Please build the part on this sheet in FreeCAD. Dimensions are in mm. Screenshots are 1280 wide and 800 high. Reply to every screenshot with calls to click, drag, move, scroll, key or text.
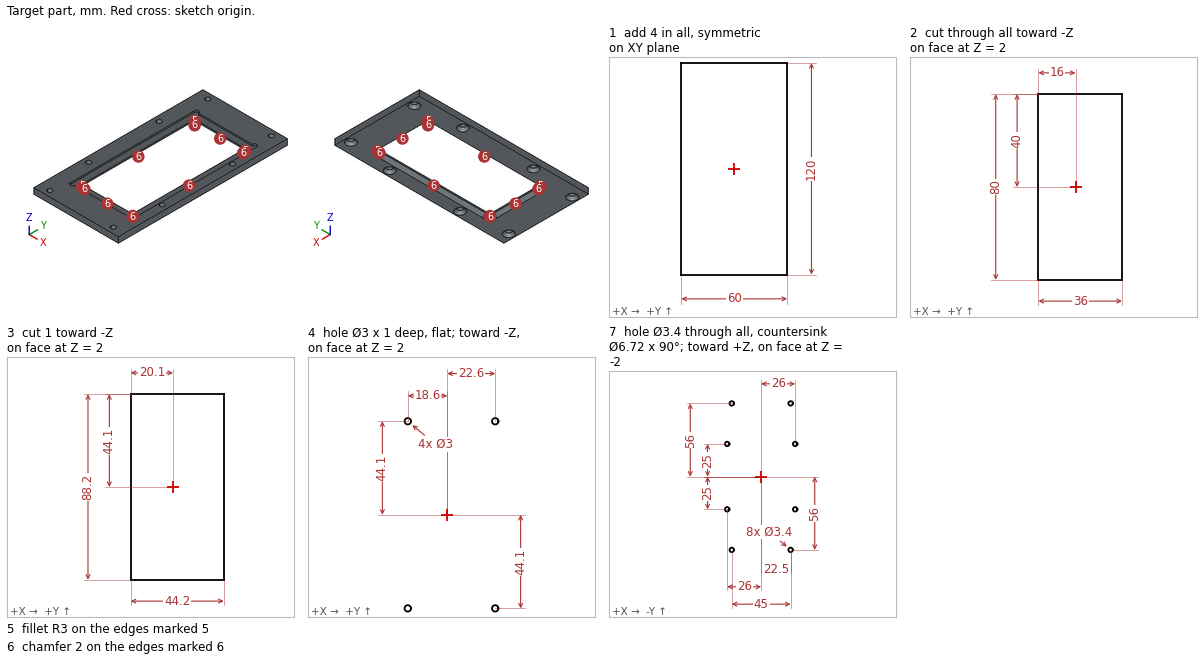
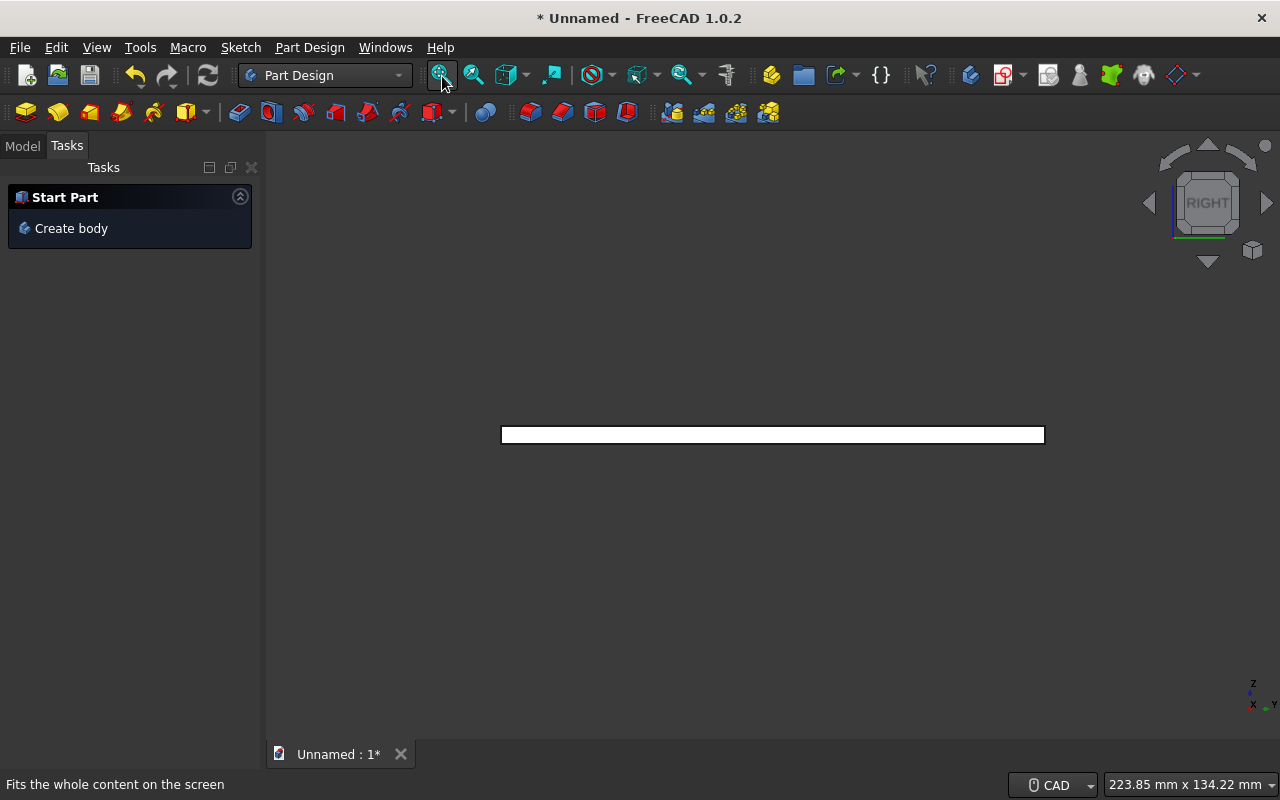
scroll(592, 436, up, 6)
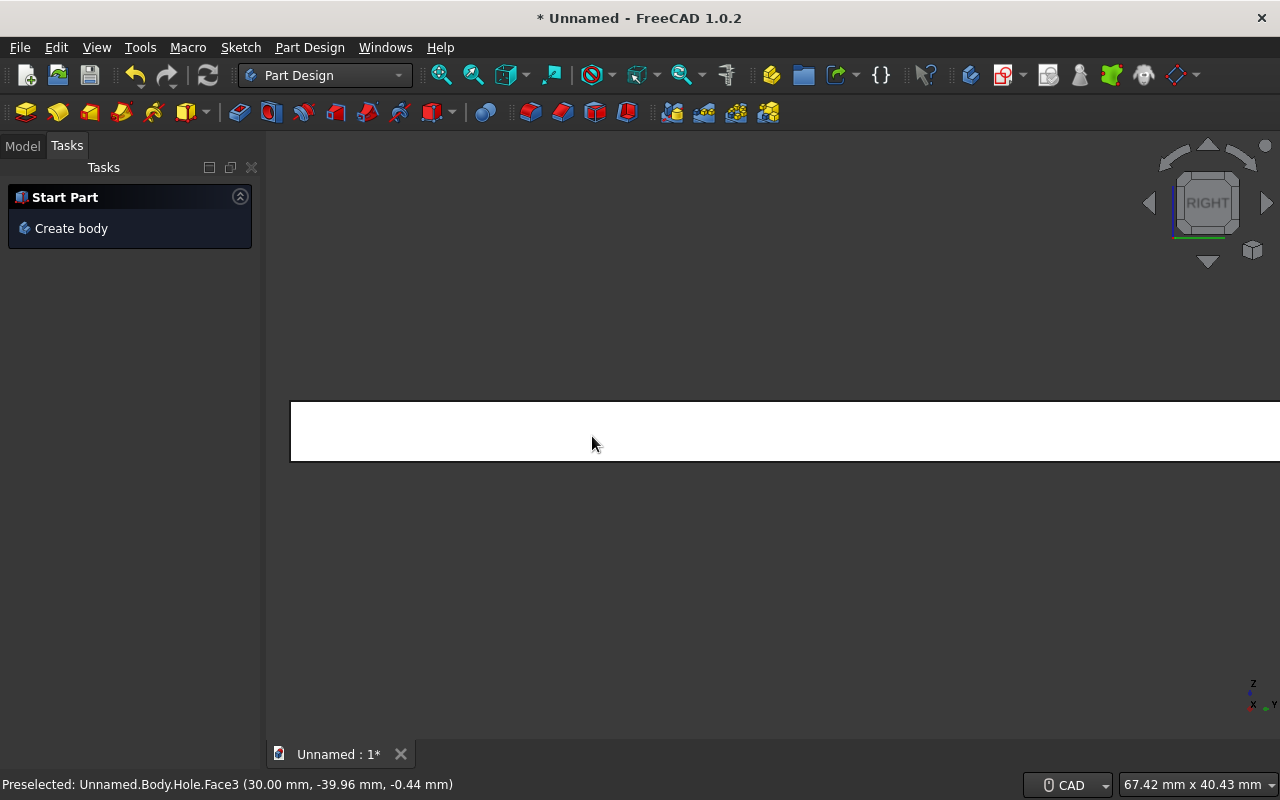
click(442, 76)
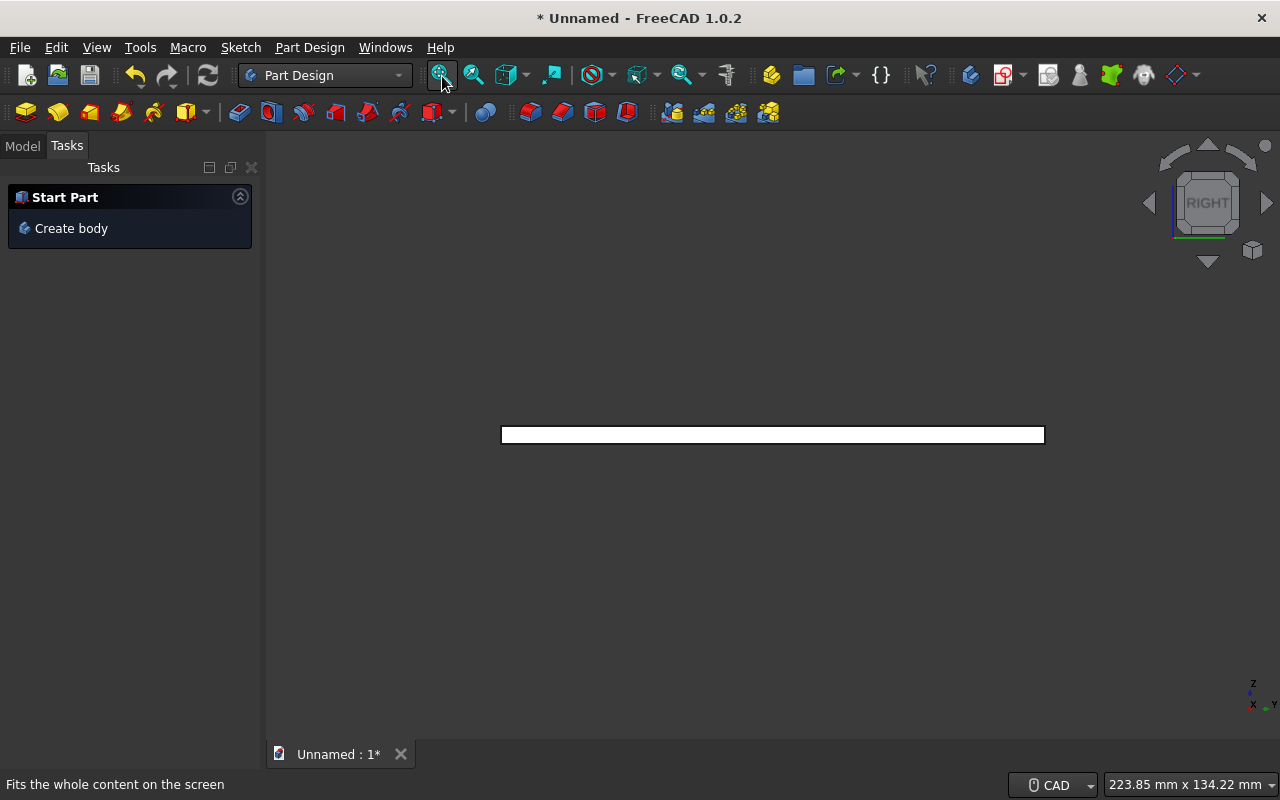
key(5)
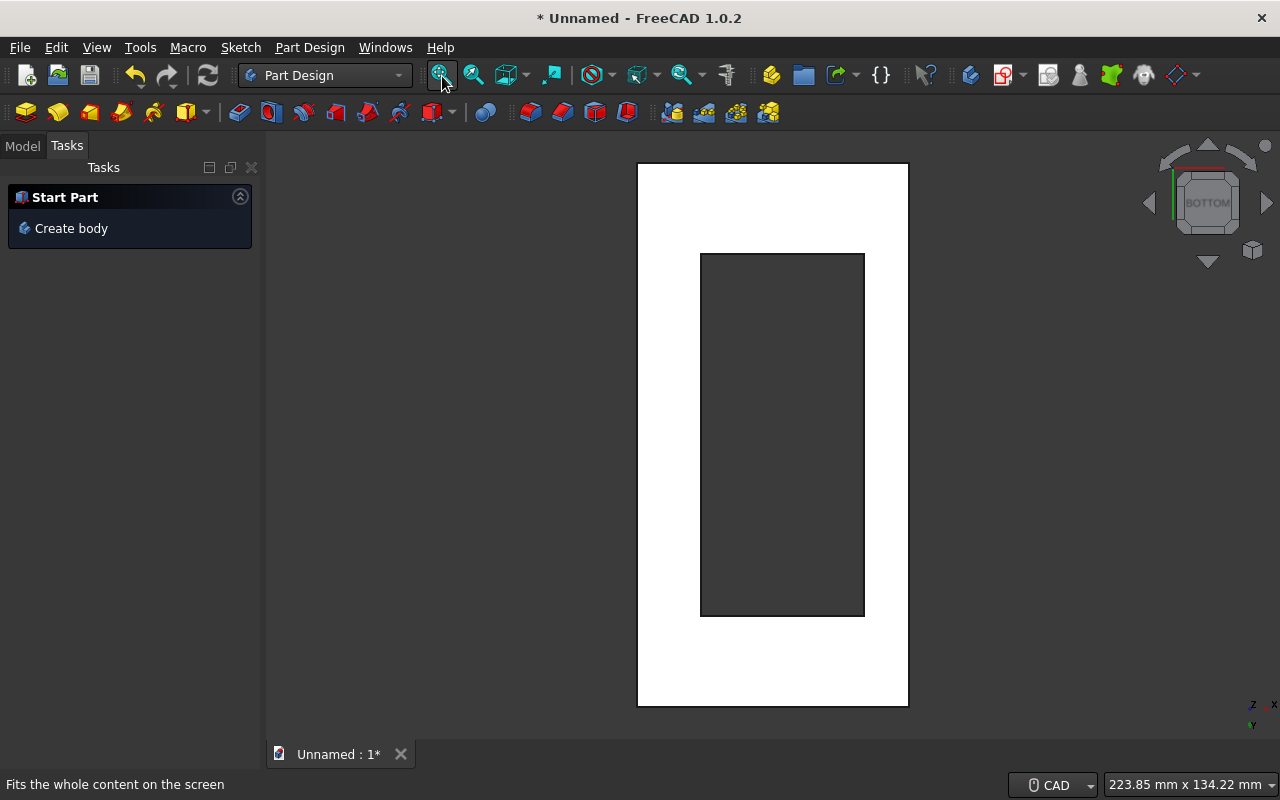
scroll(701, 253, up, 6)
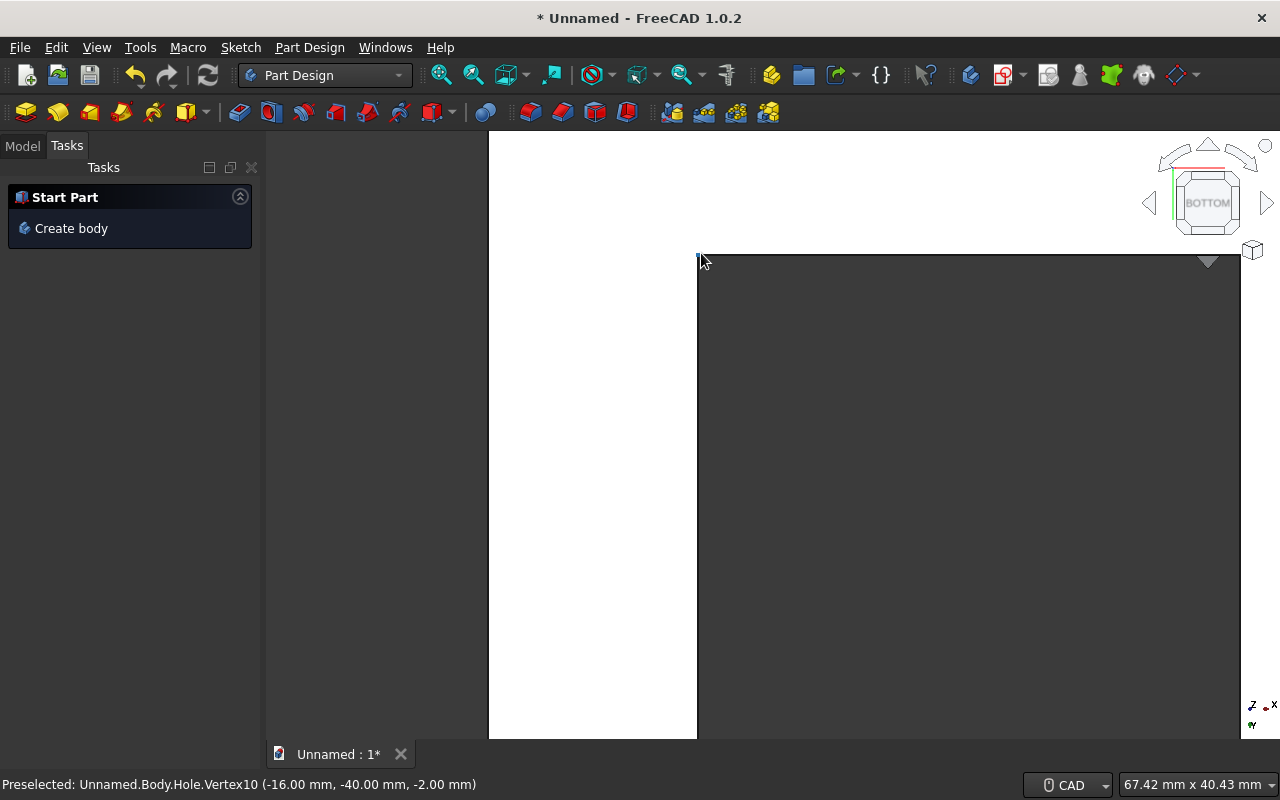
click(442, 76)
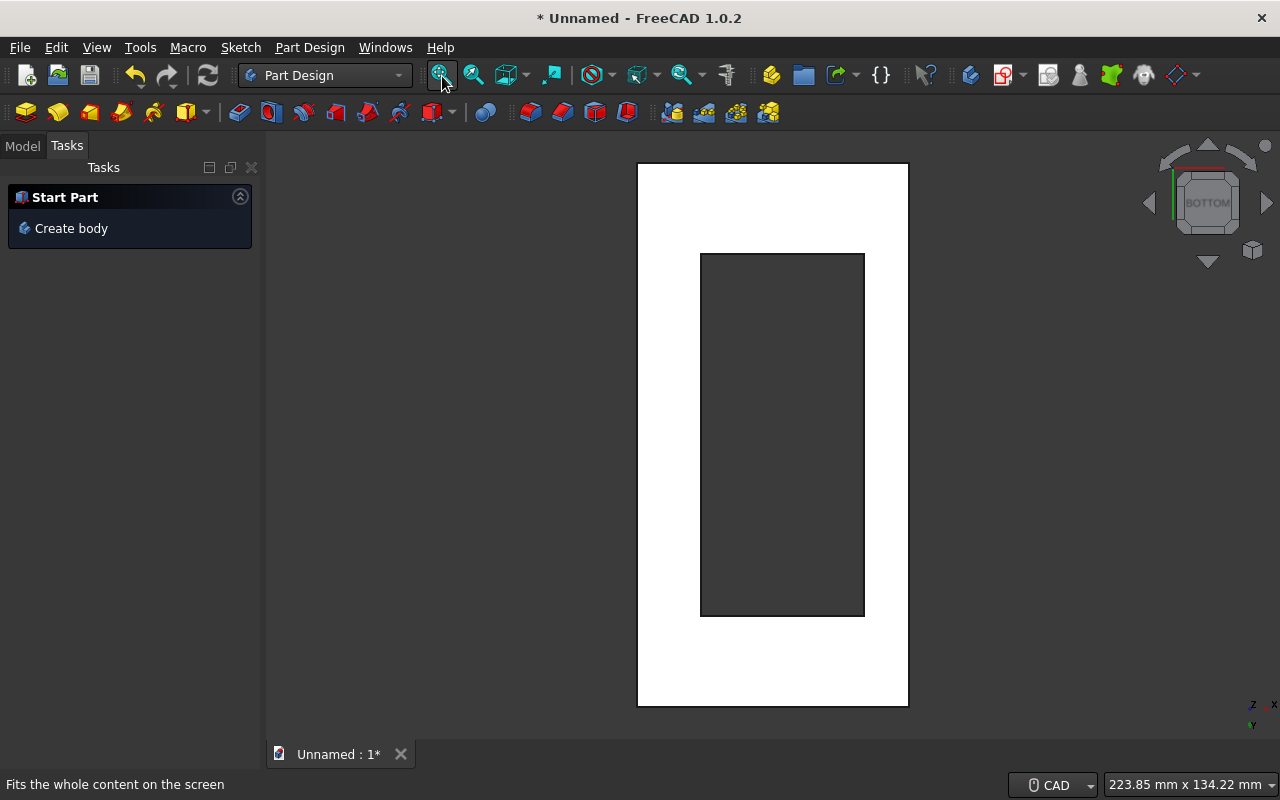
key(4)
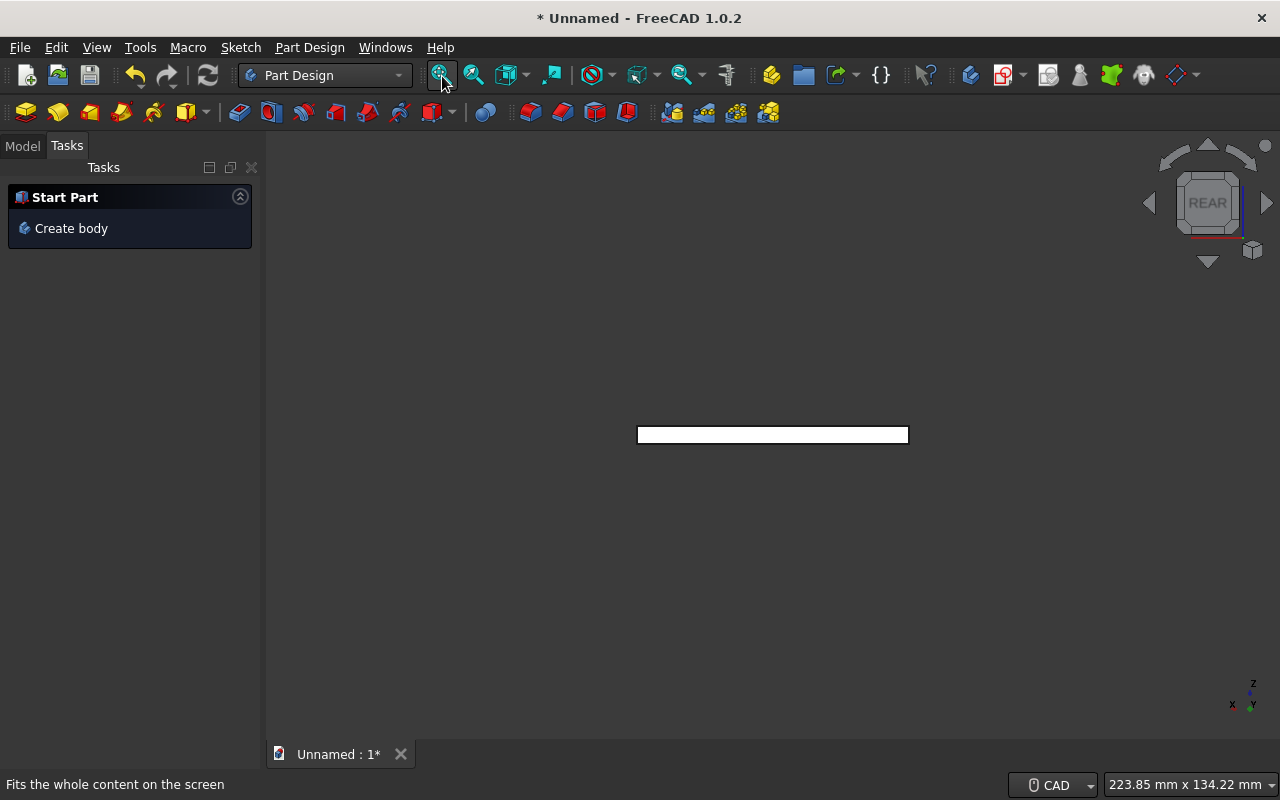
click(442, 76)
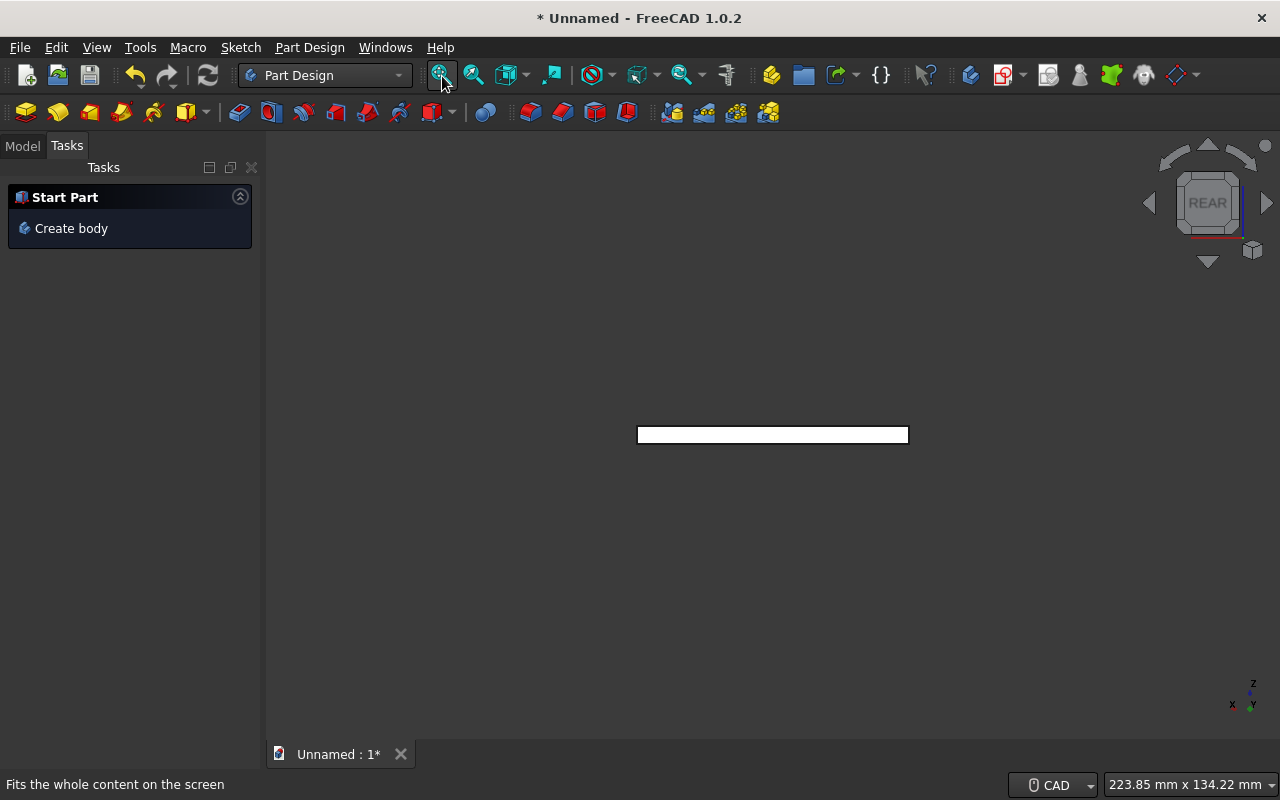
scroll(845, 436, up, 6)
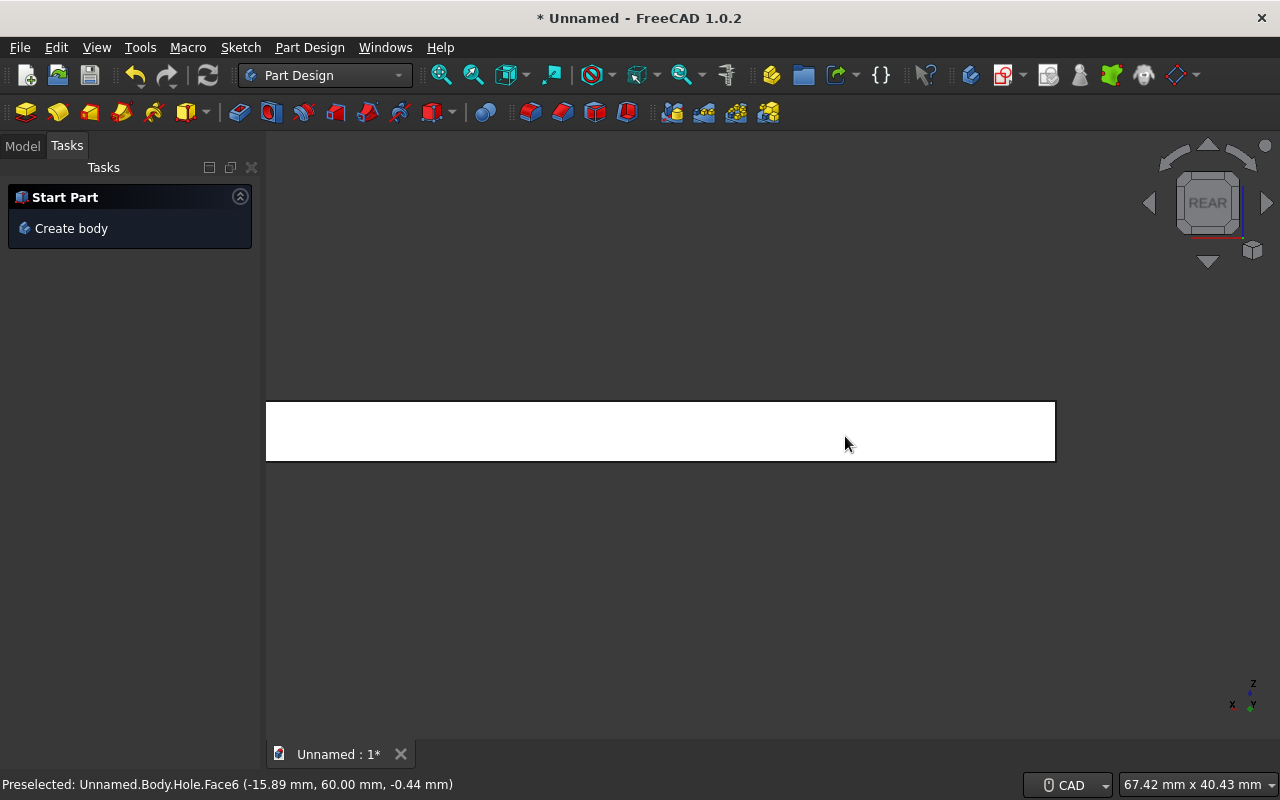
click(442, 76)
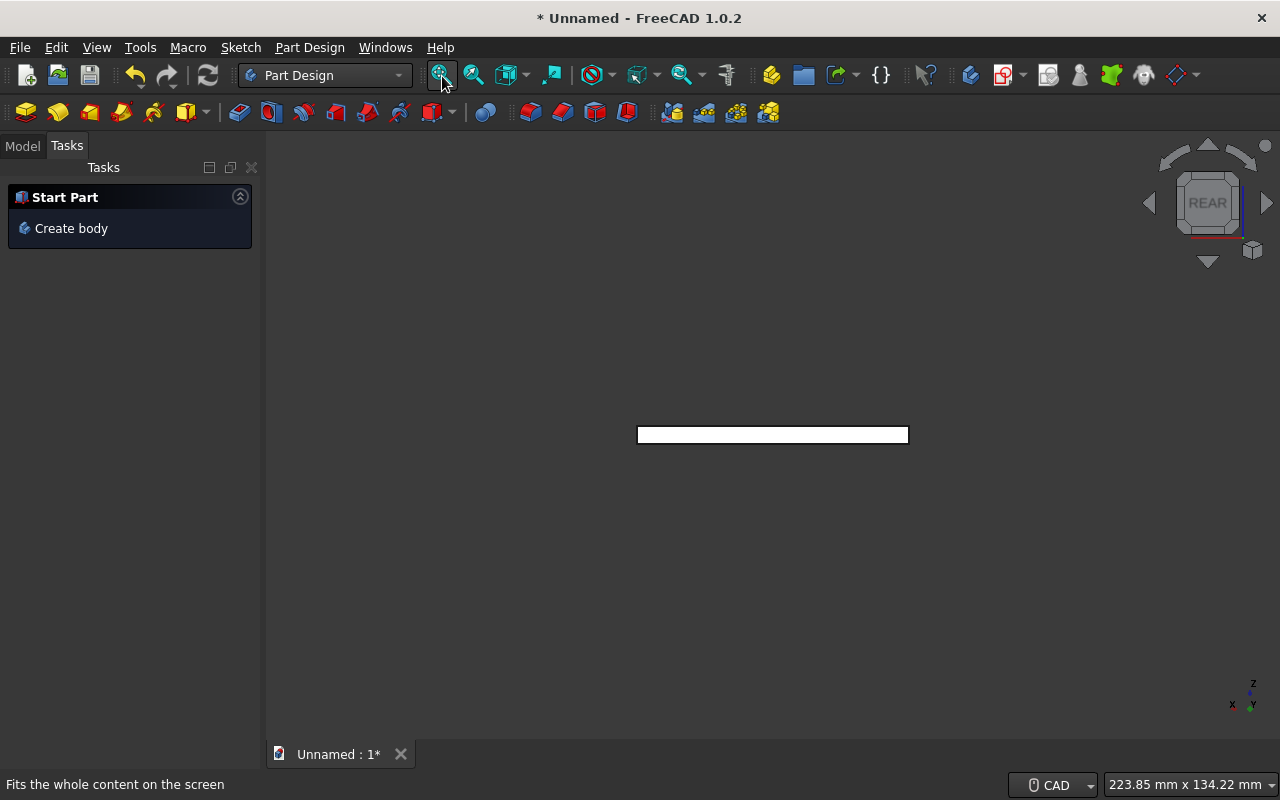
key(6)